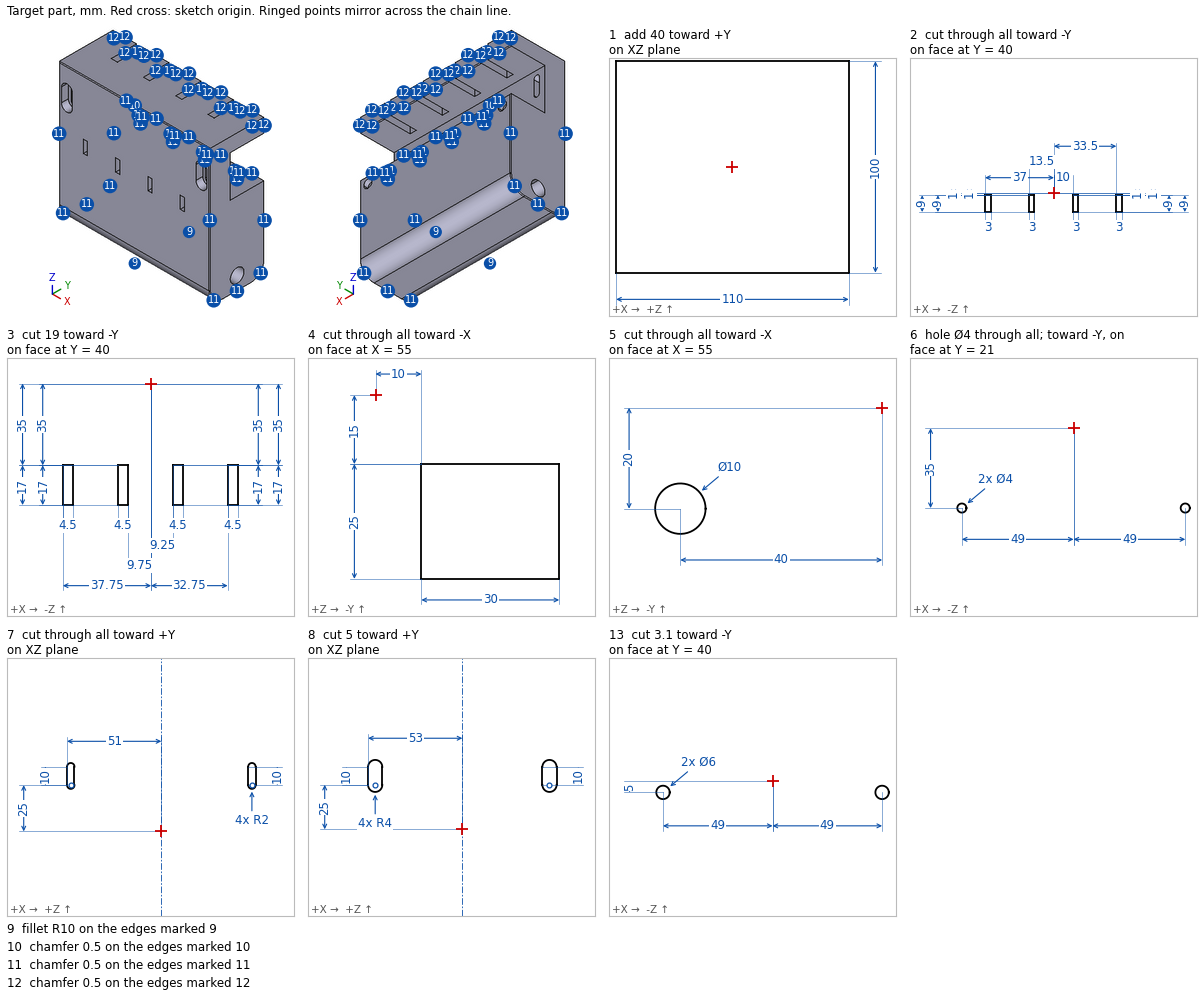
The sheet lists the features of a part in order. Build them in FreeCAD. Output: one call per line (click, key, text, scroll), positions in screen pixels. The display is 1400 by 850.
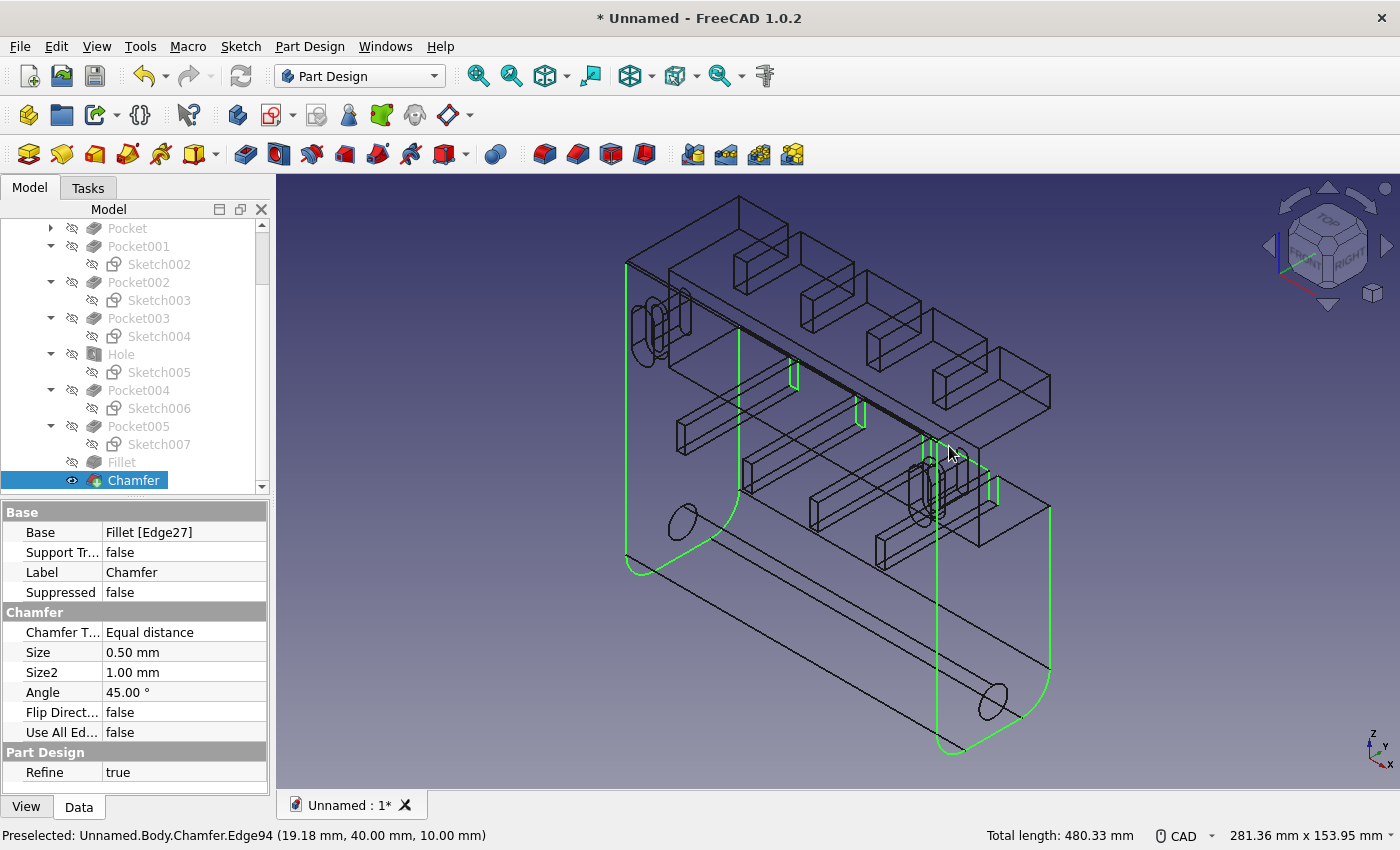
click(991, 500, ctrl)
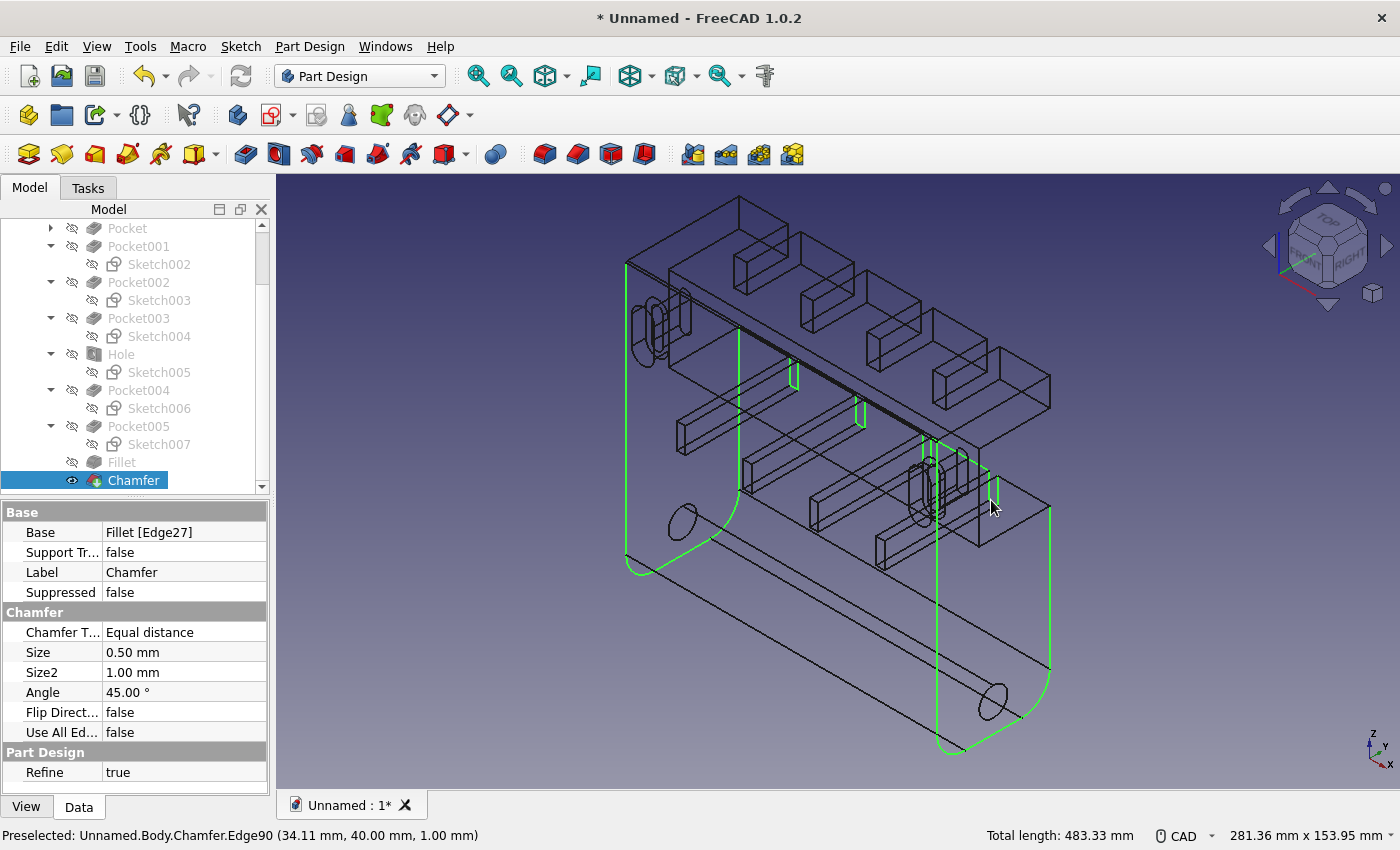
click(1024, 490, ctrl)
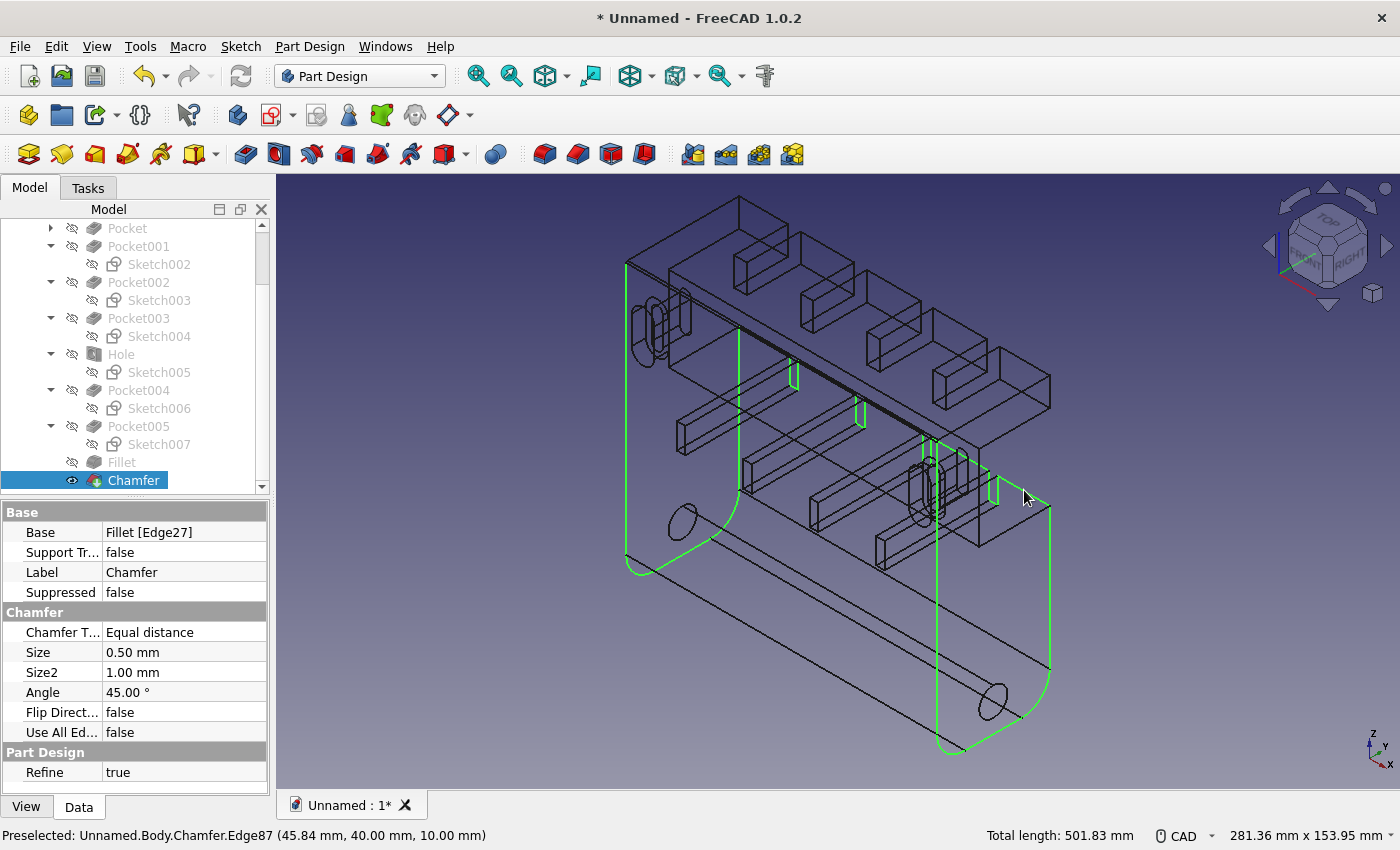
key(2)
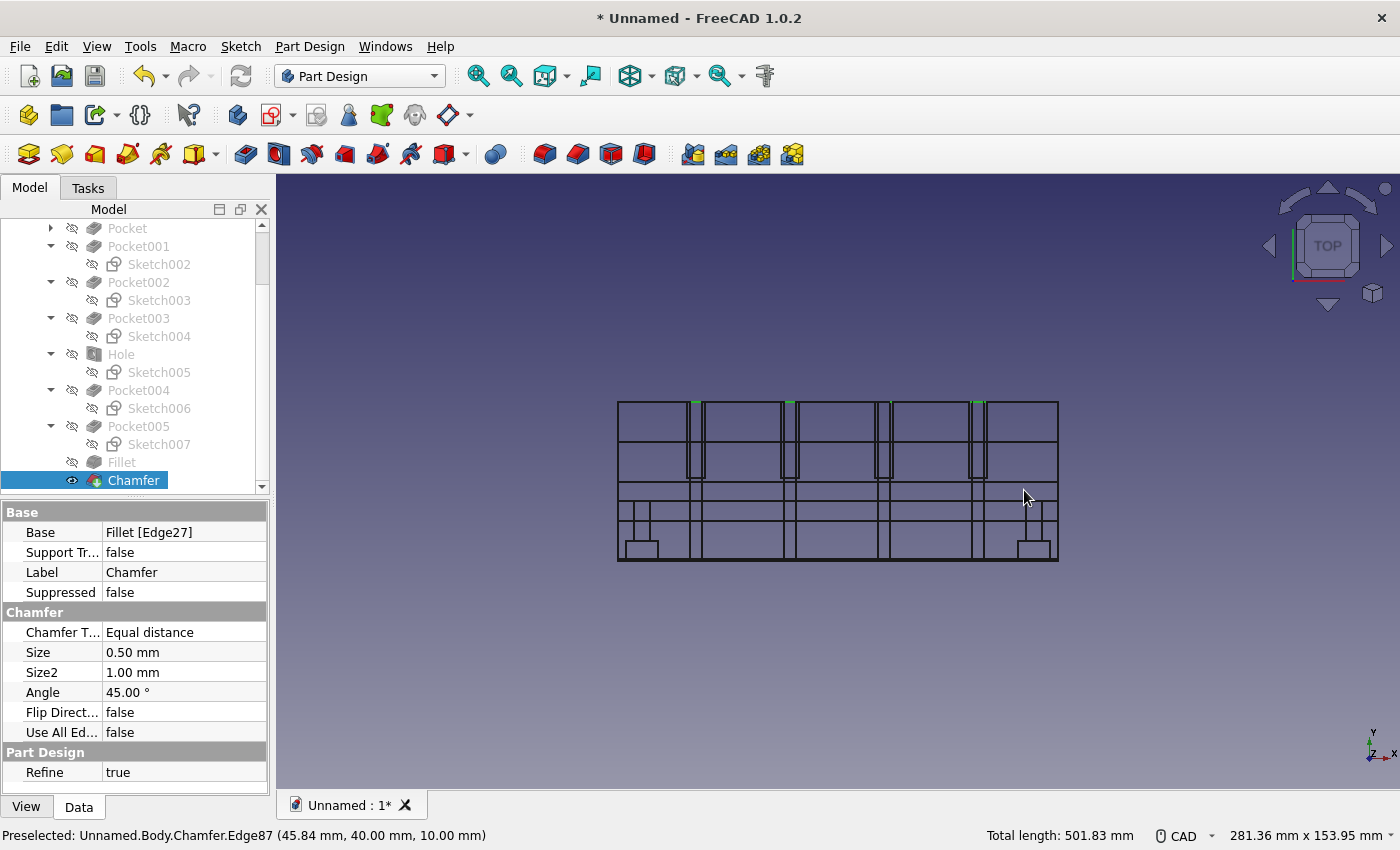
key(v)
key(f)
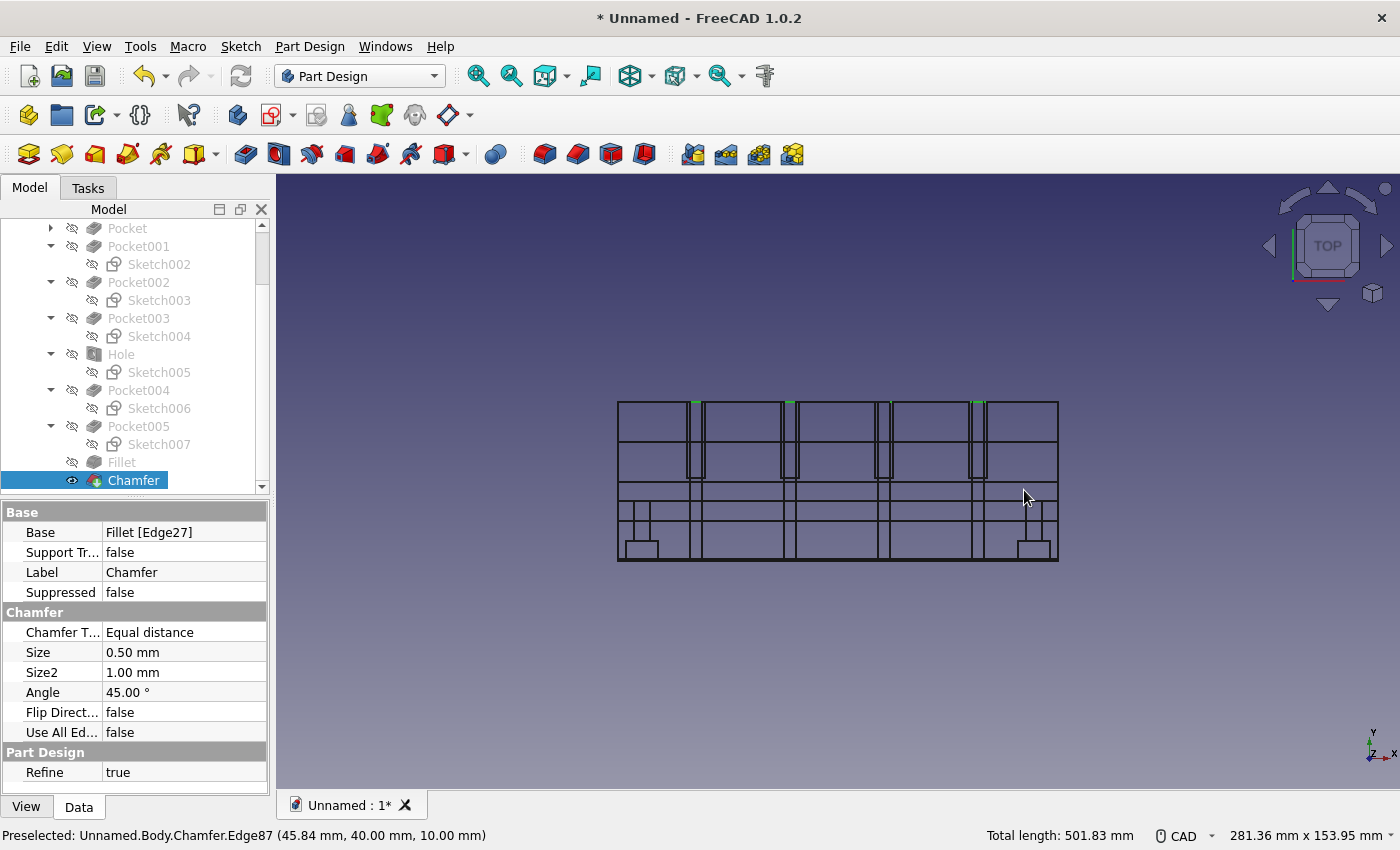
key(1)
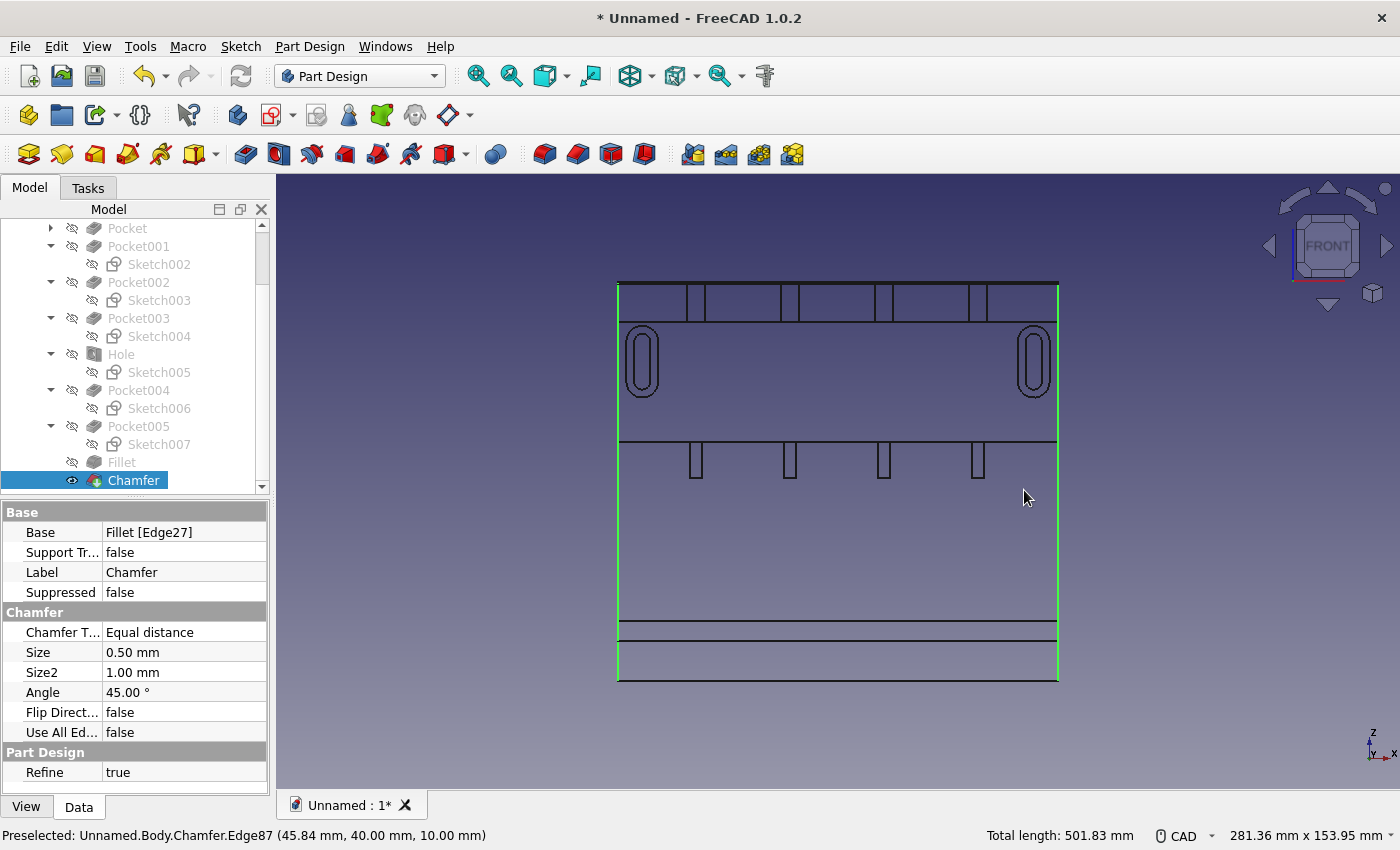
key(3)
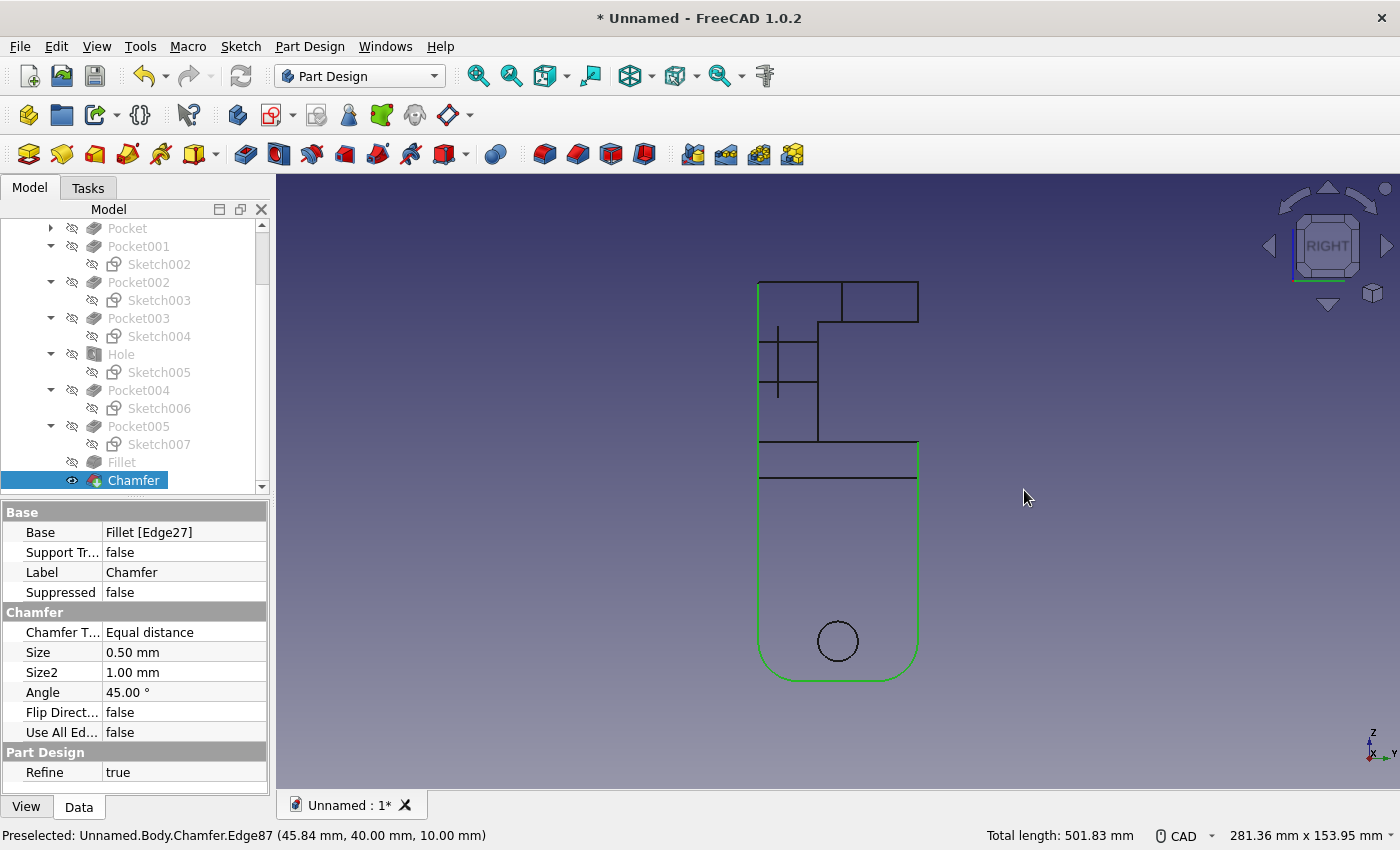
key(5)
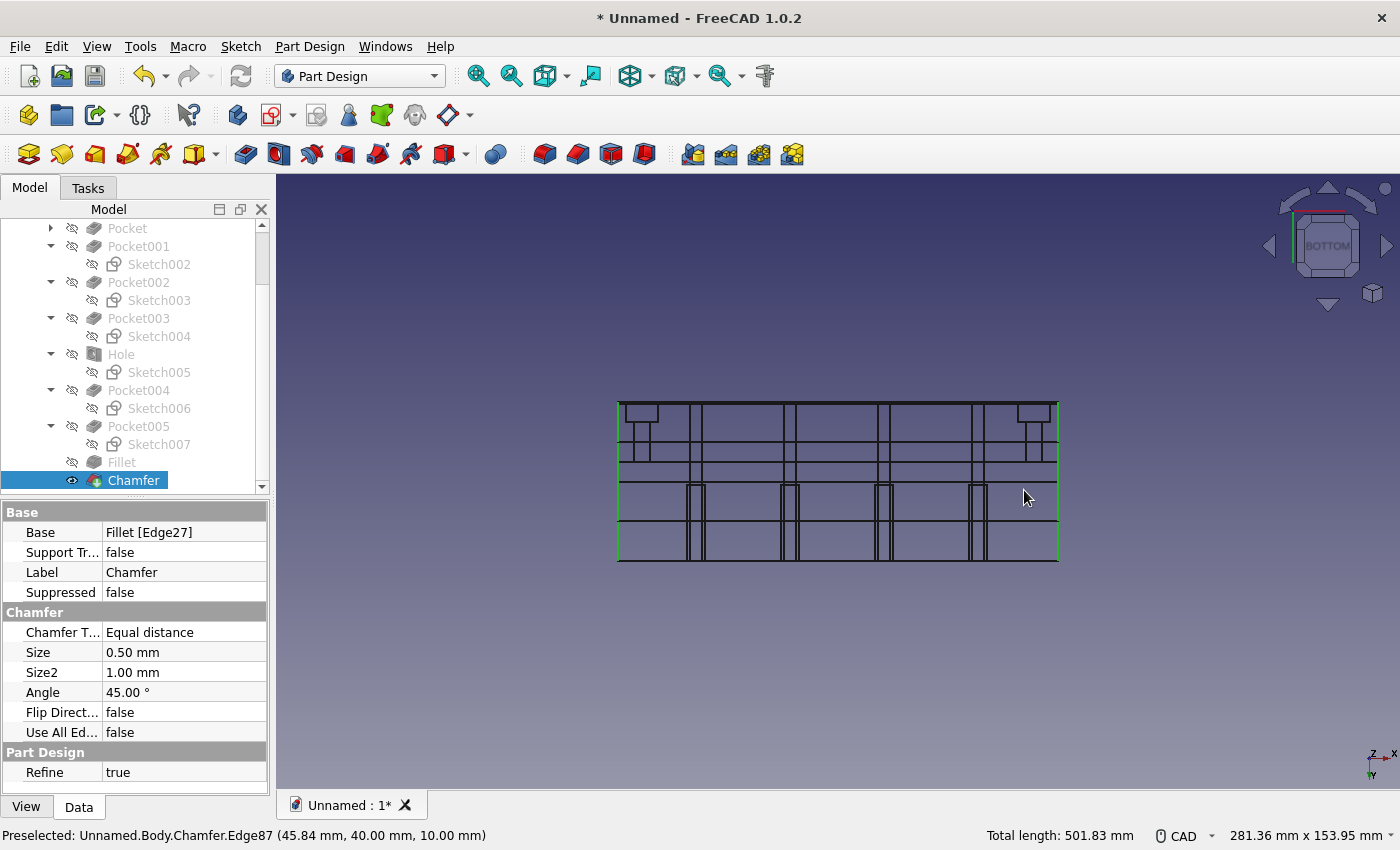
key(v)
key(f)